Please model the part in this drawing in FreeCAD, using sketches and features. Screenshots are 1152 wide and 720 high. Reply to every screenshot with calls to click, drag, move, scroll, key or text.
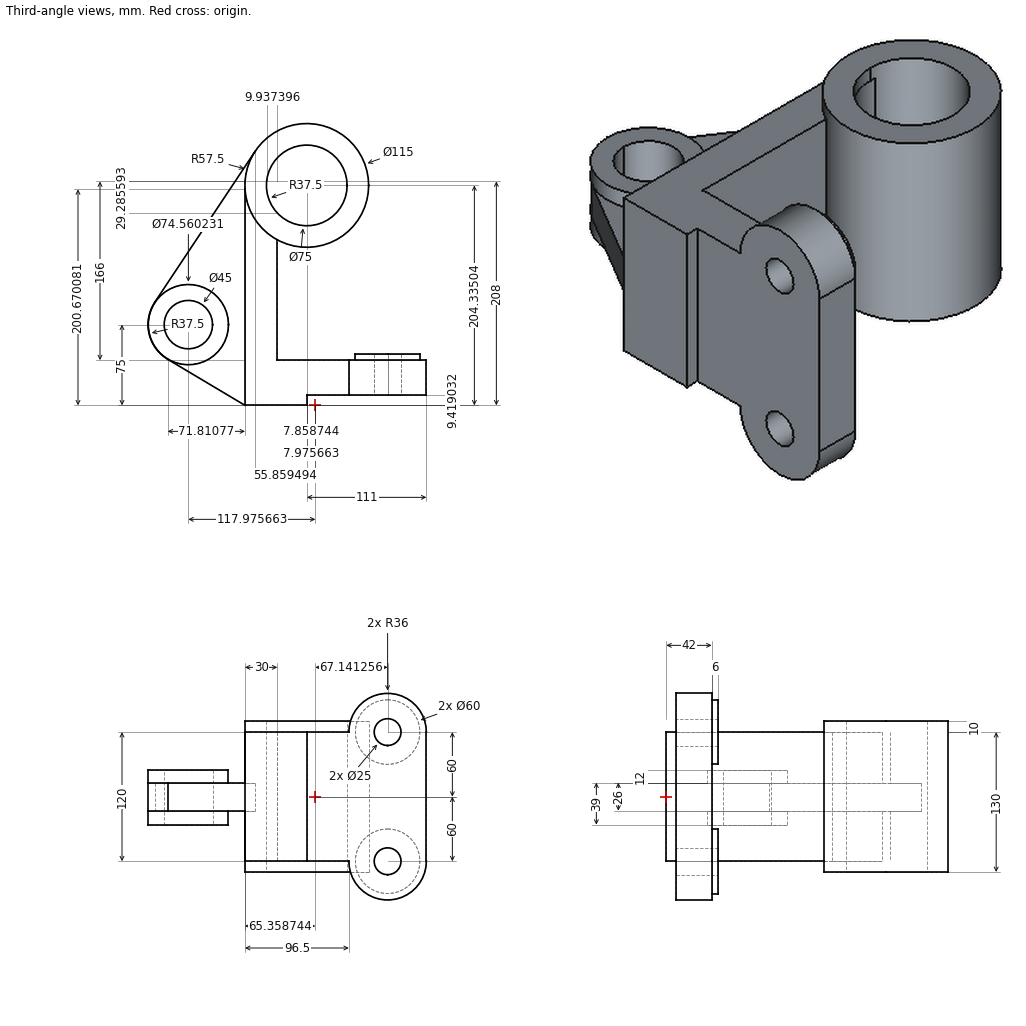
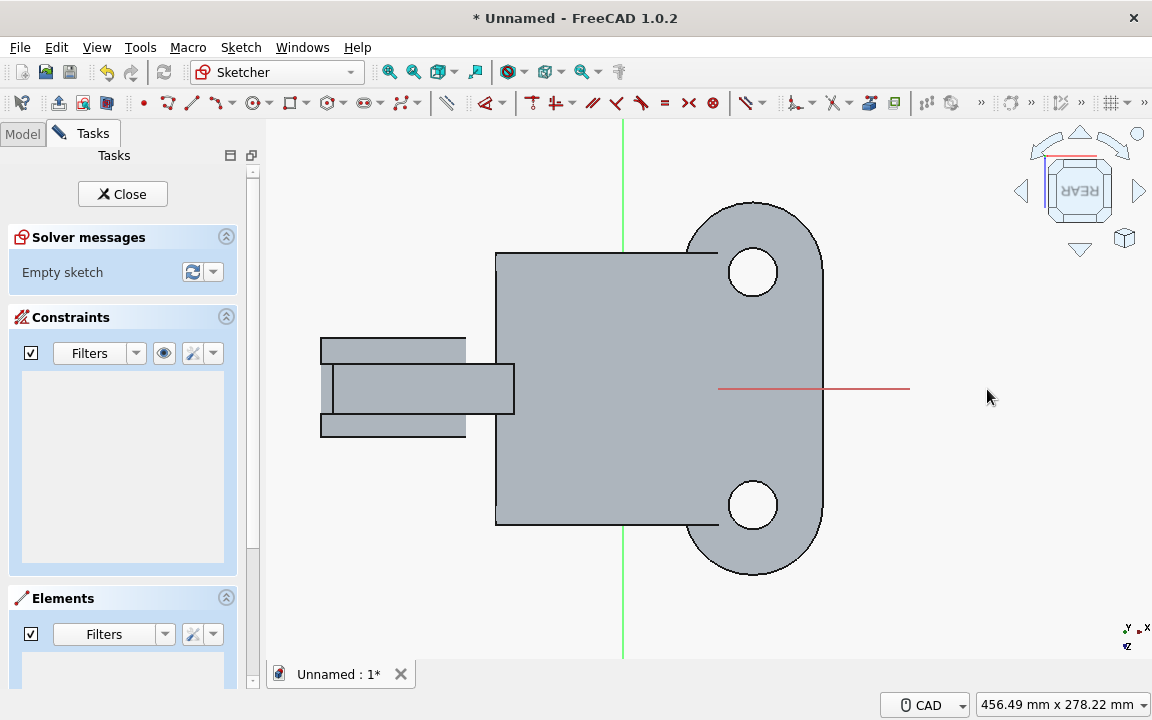
click(254, 104)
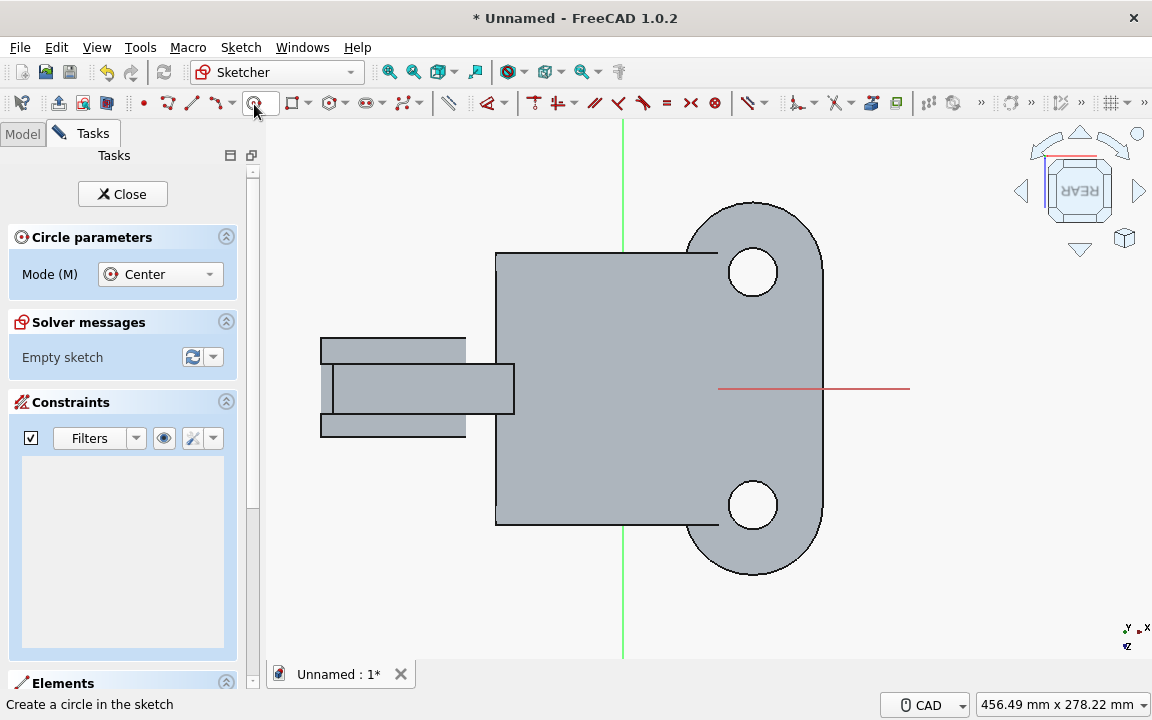
click(753, 505)
move(794, 464)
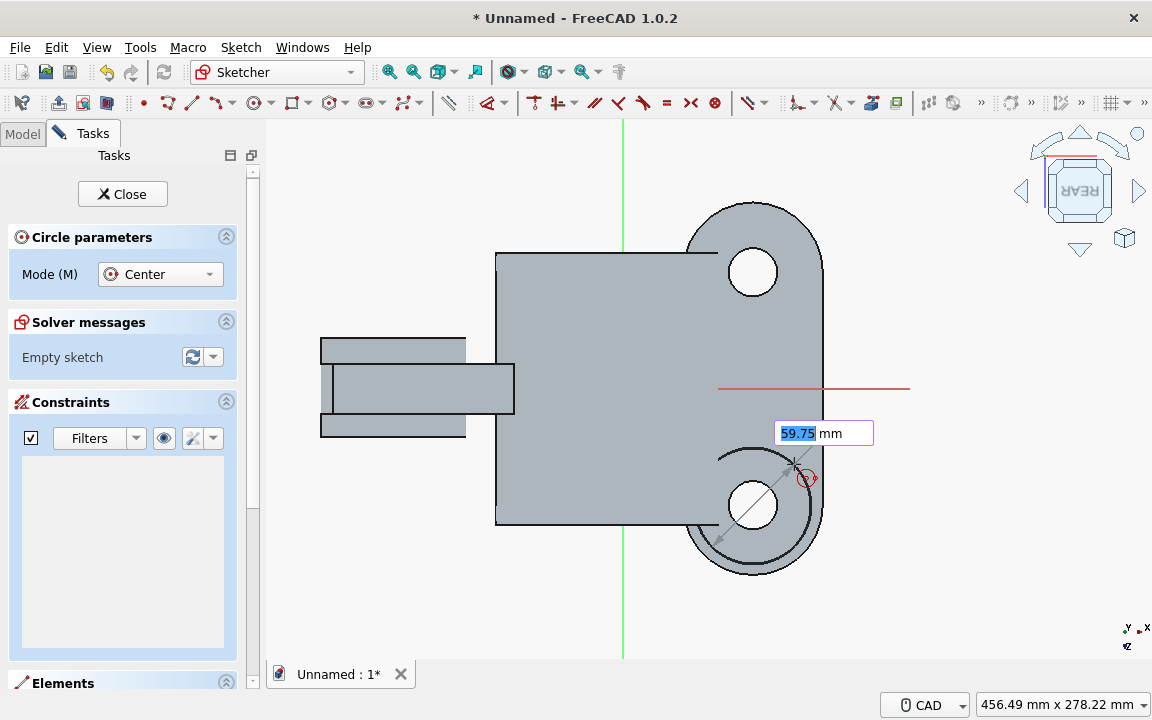
text(60)
key(Return)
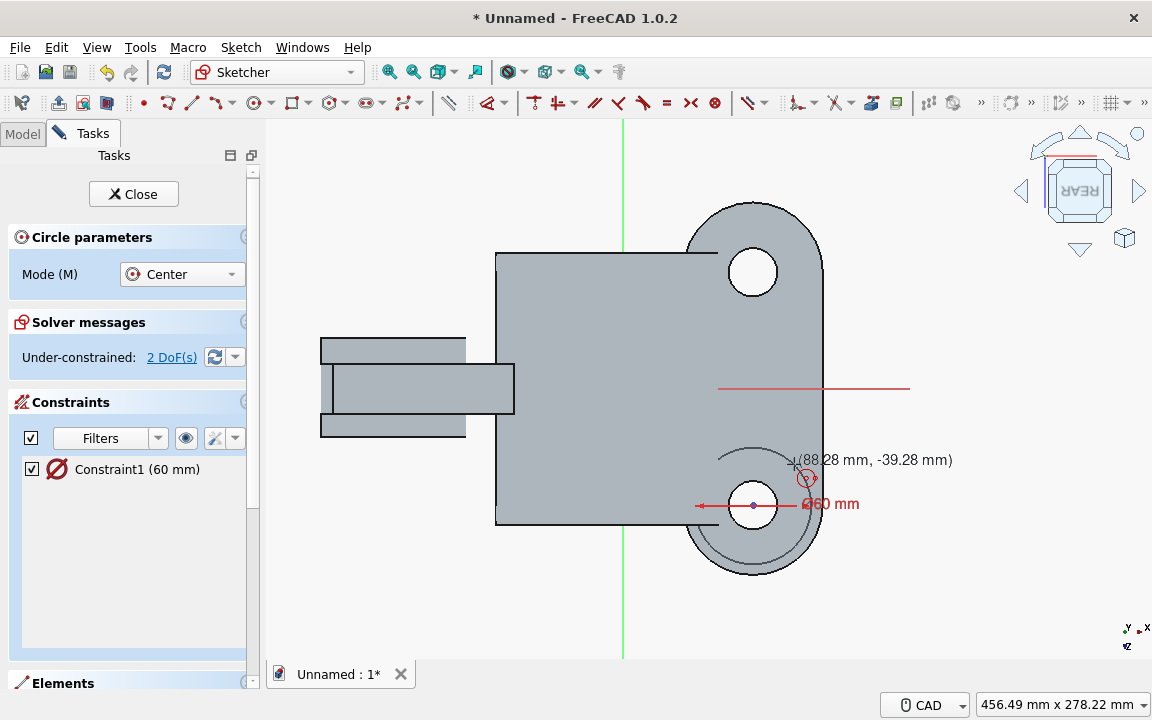
click(753, 272)
move(794, 231)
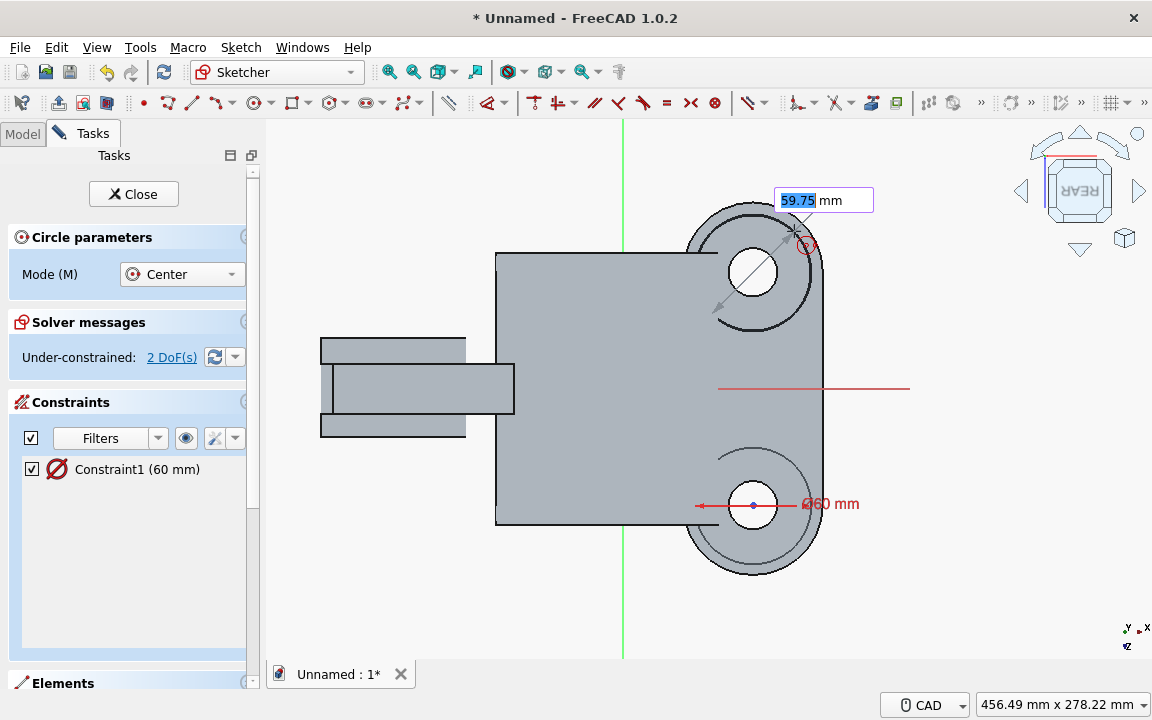
text(60)
key(Return)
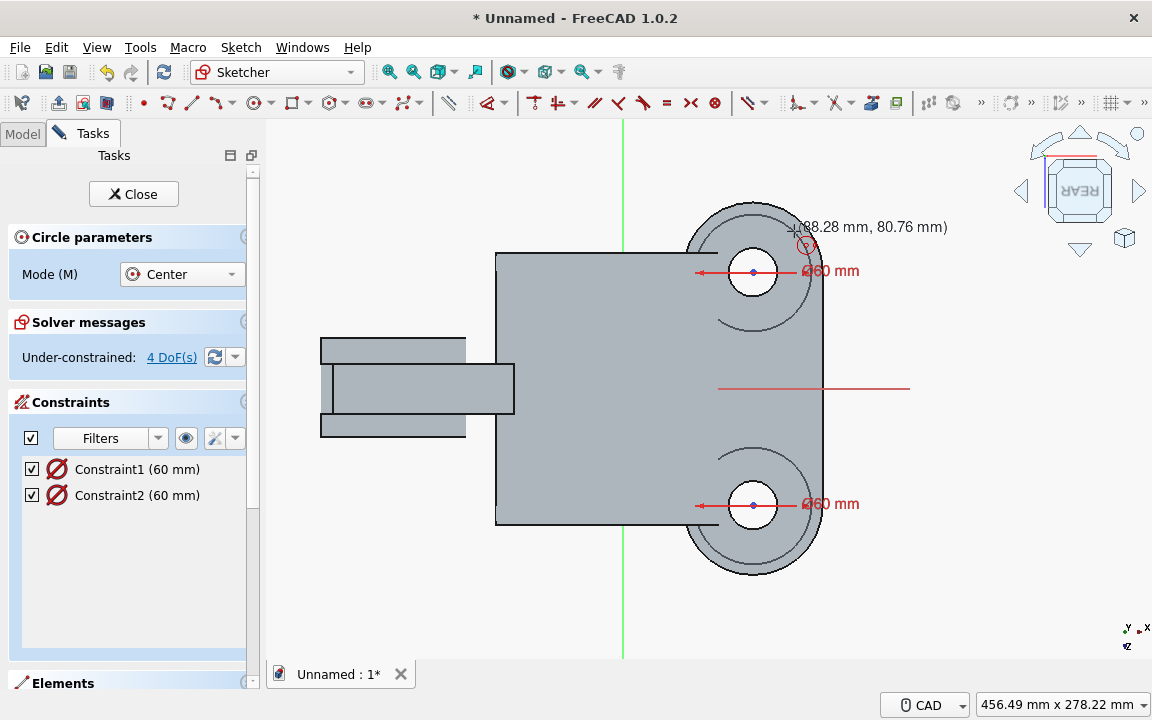
click(753, 506)
move(770, 488)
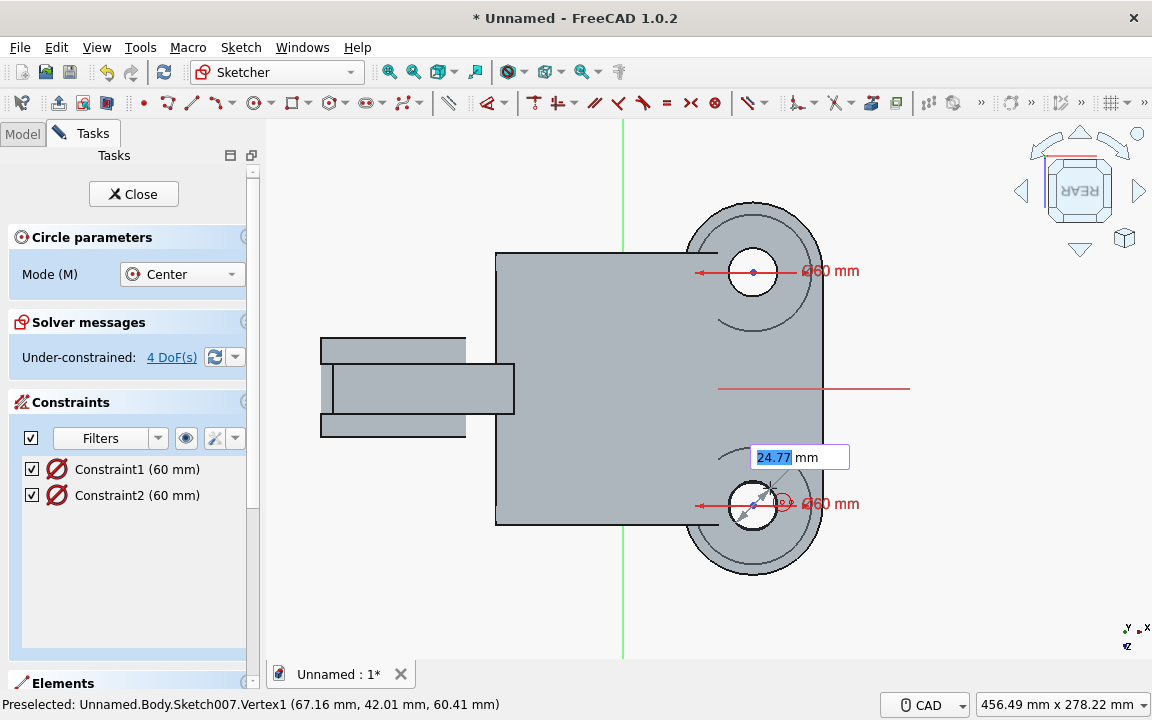
text(25)
key(Return)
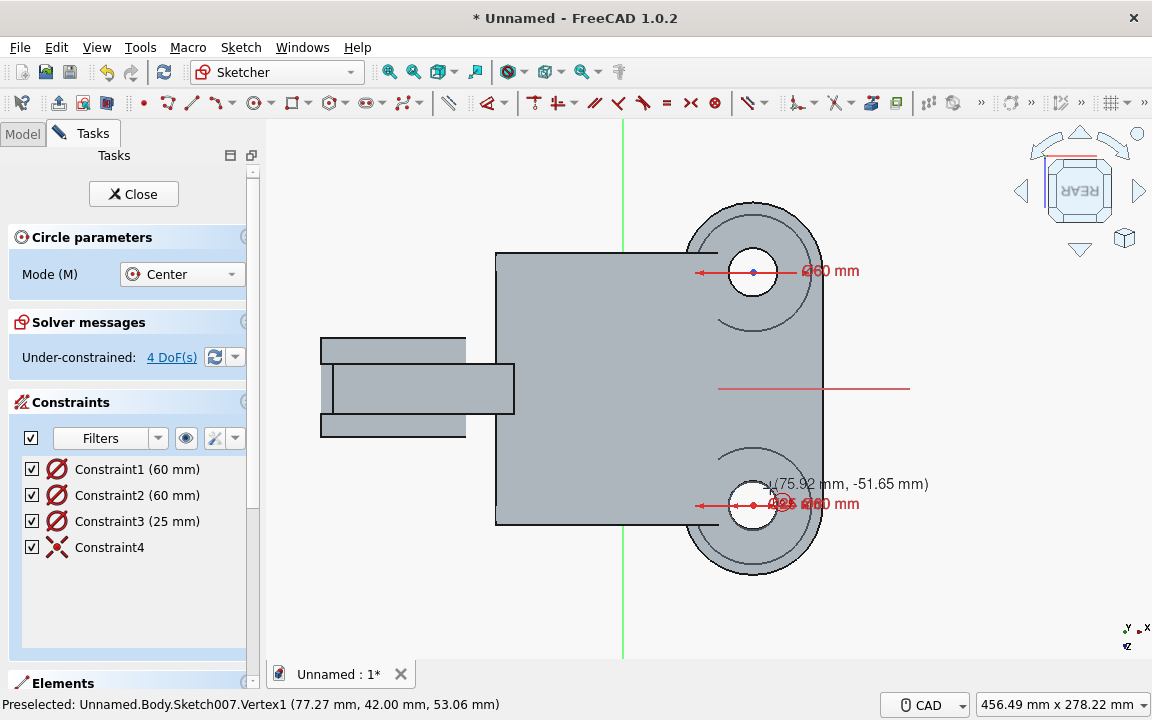
click(753, 273)
move(770, 255)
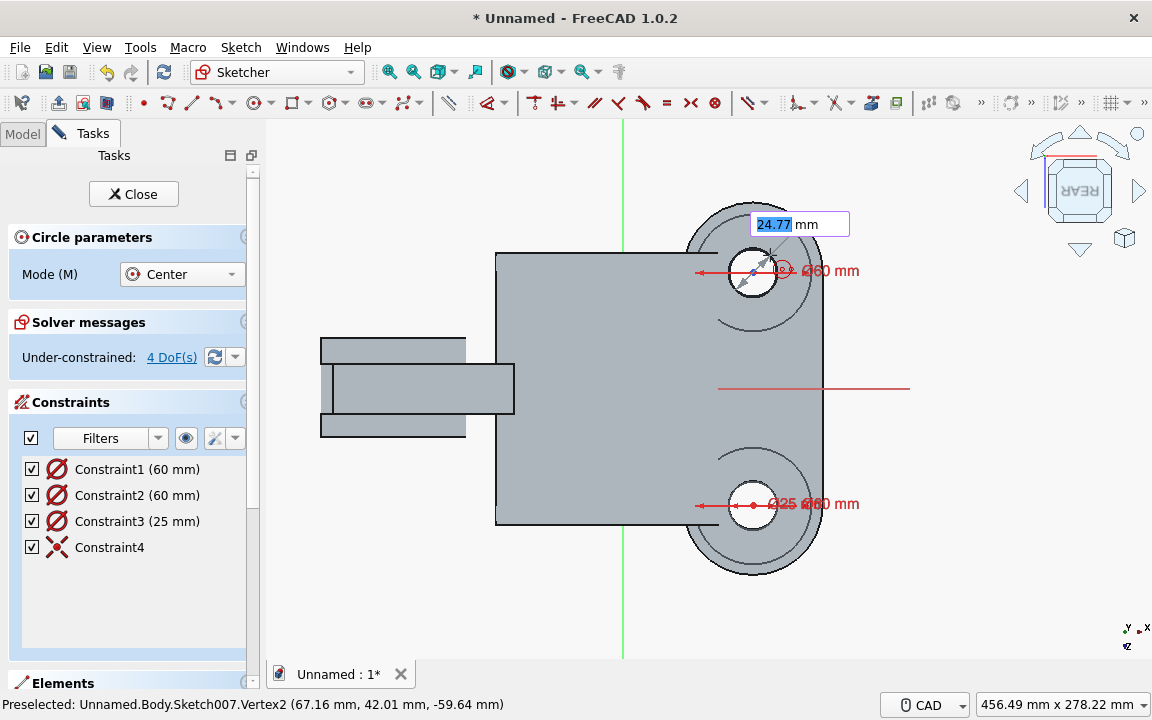
text(25)
key(Return)
key(Escape)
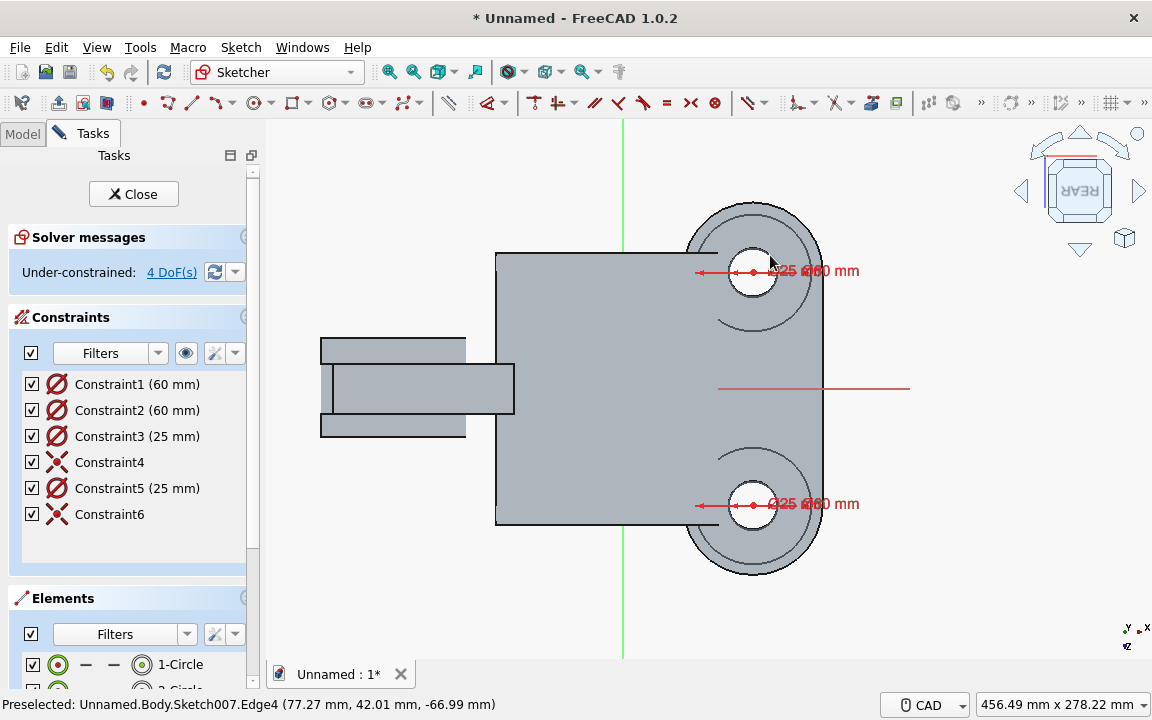
click(753, 506)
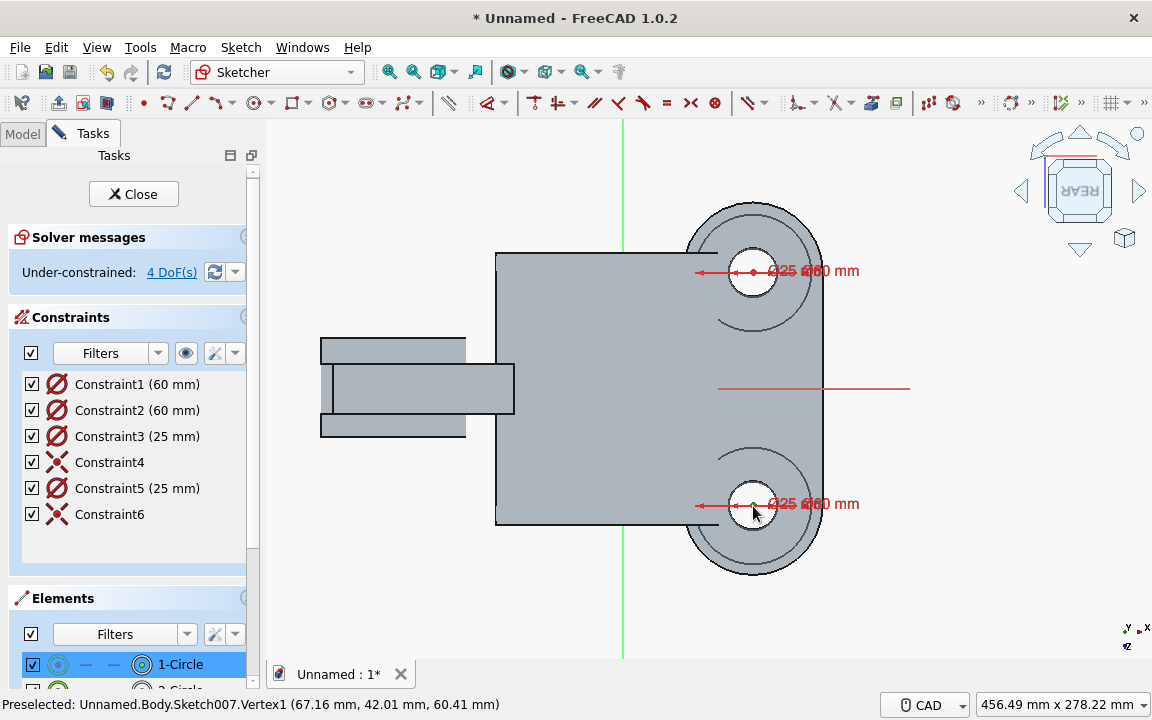
click(753, 273)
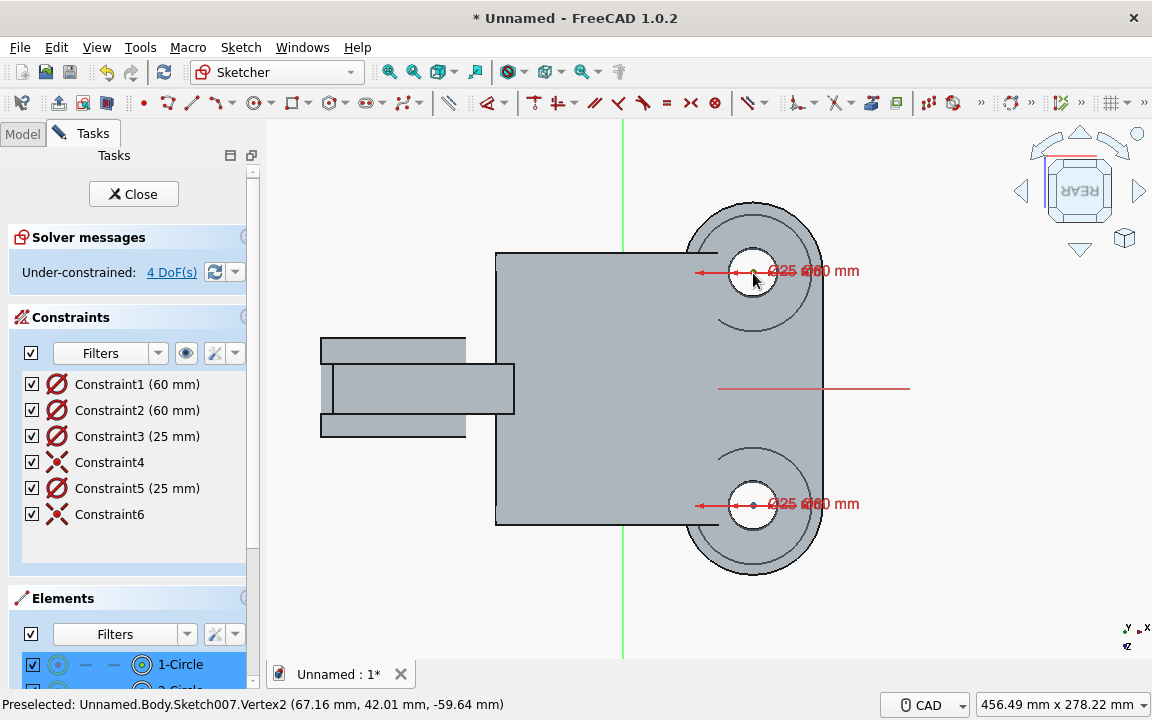
click(576, 104)